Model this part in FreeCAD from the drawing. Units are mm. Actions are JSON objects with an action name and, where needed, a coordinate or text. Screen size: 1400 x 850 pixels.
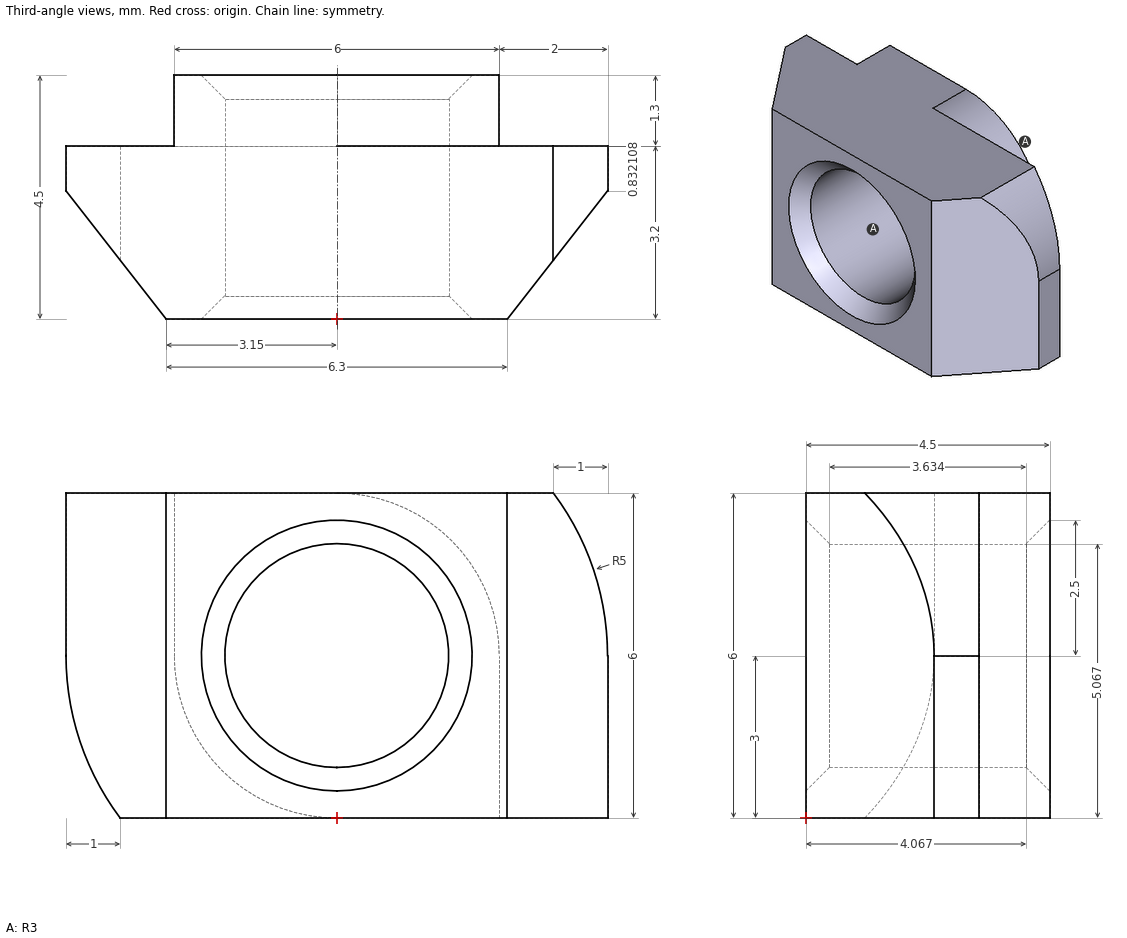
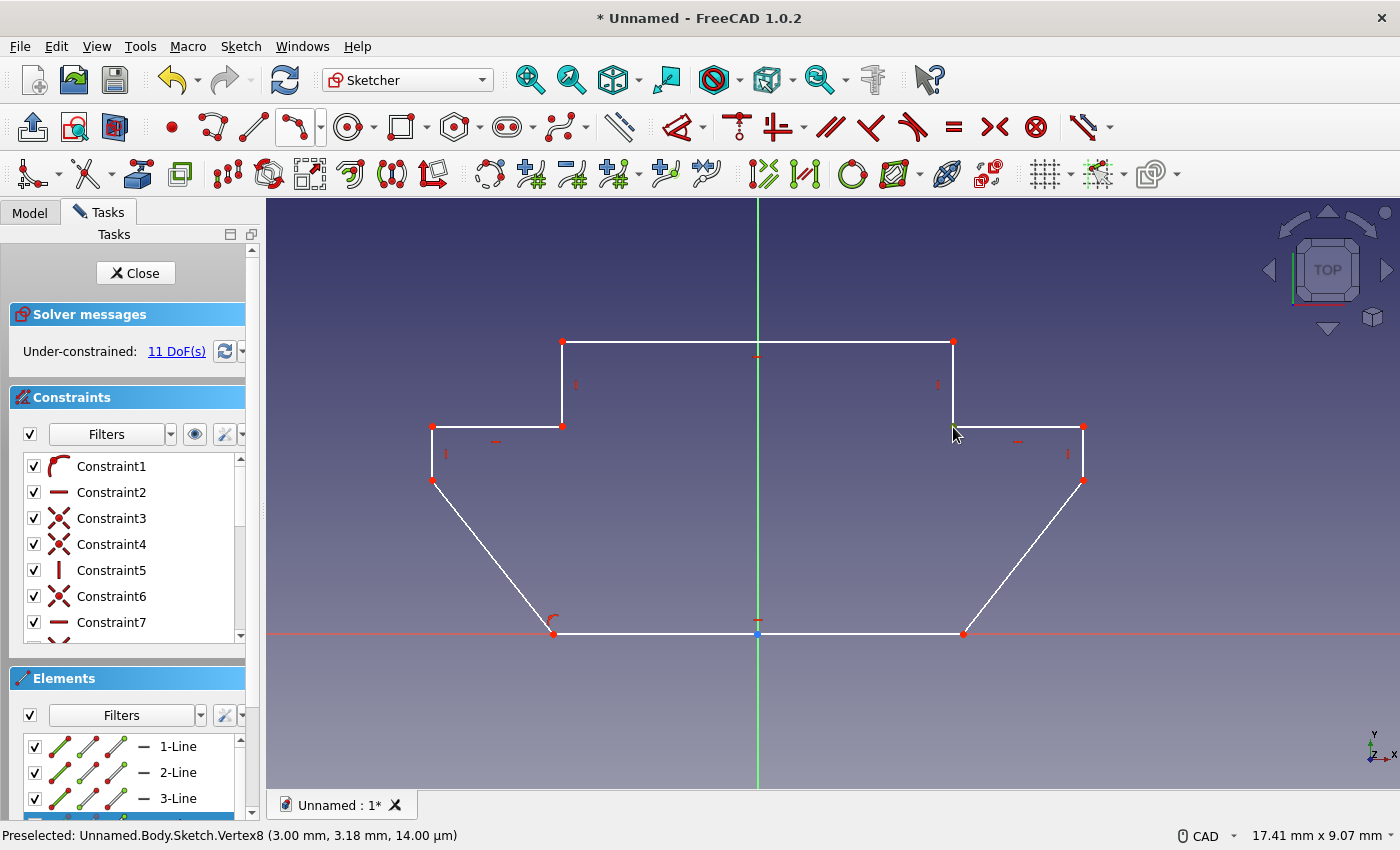
{"action": "left_click", "coordinate": [562, 427]}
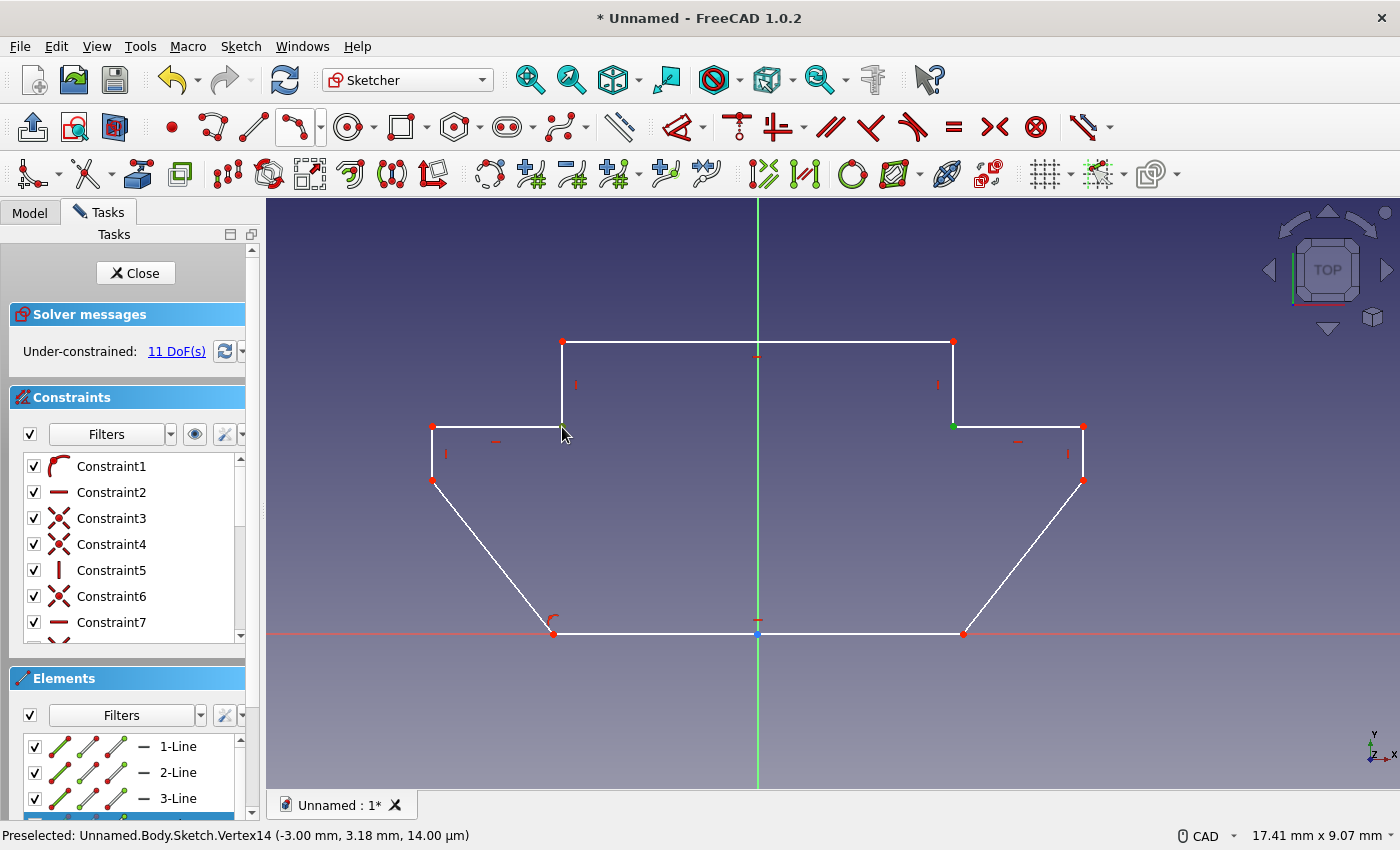
{"action": "left_click", "coordinate": [758, 723]}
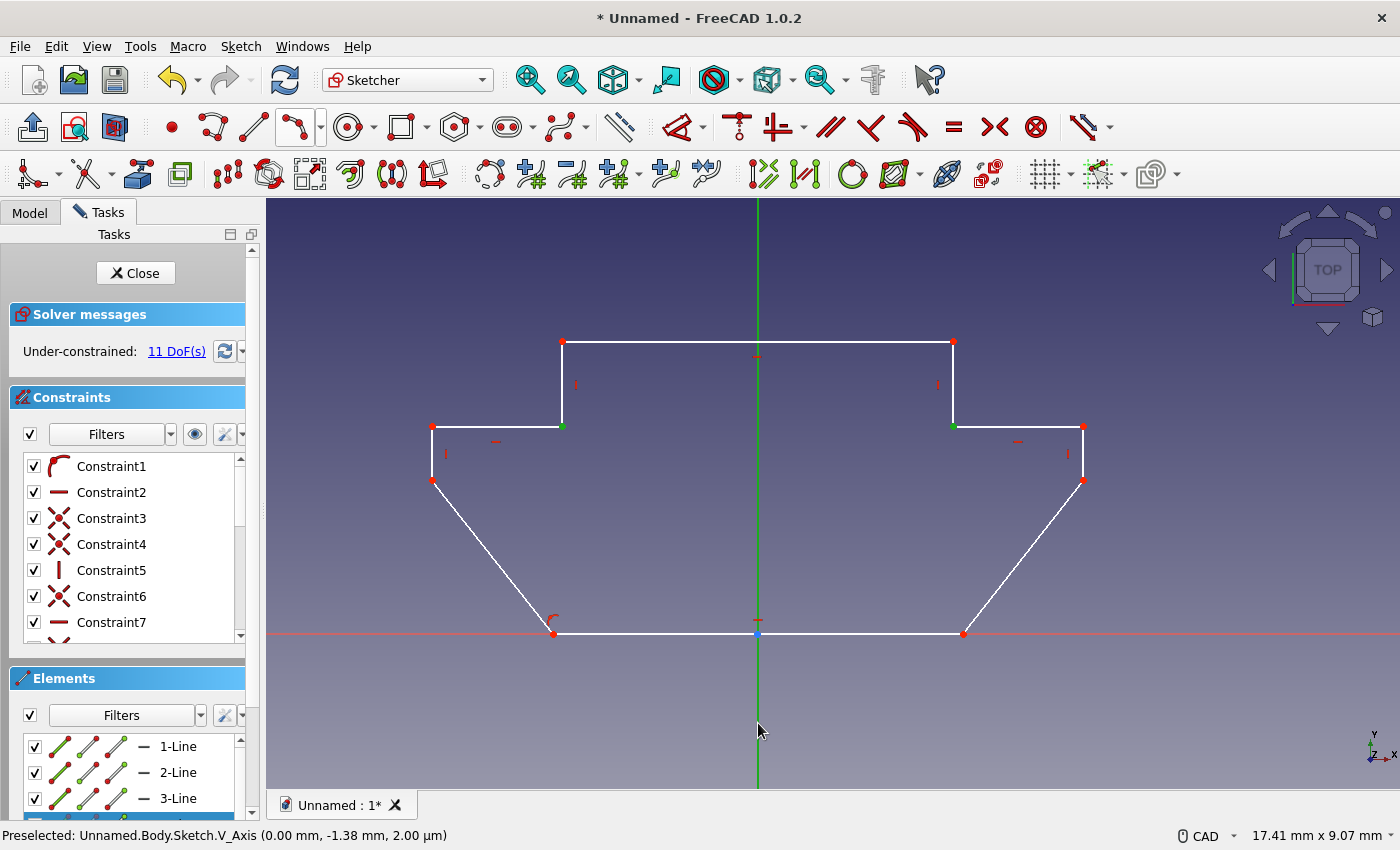
{"action": "left_click", "coordinate": [995, 128]}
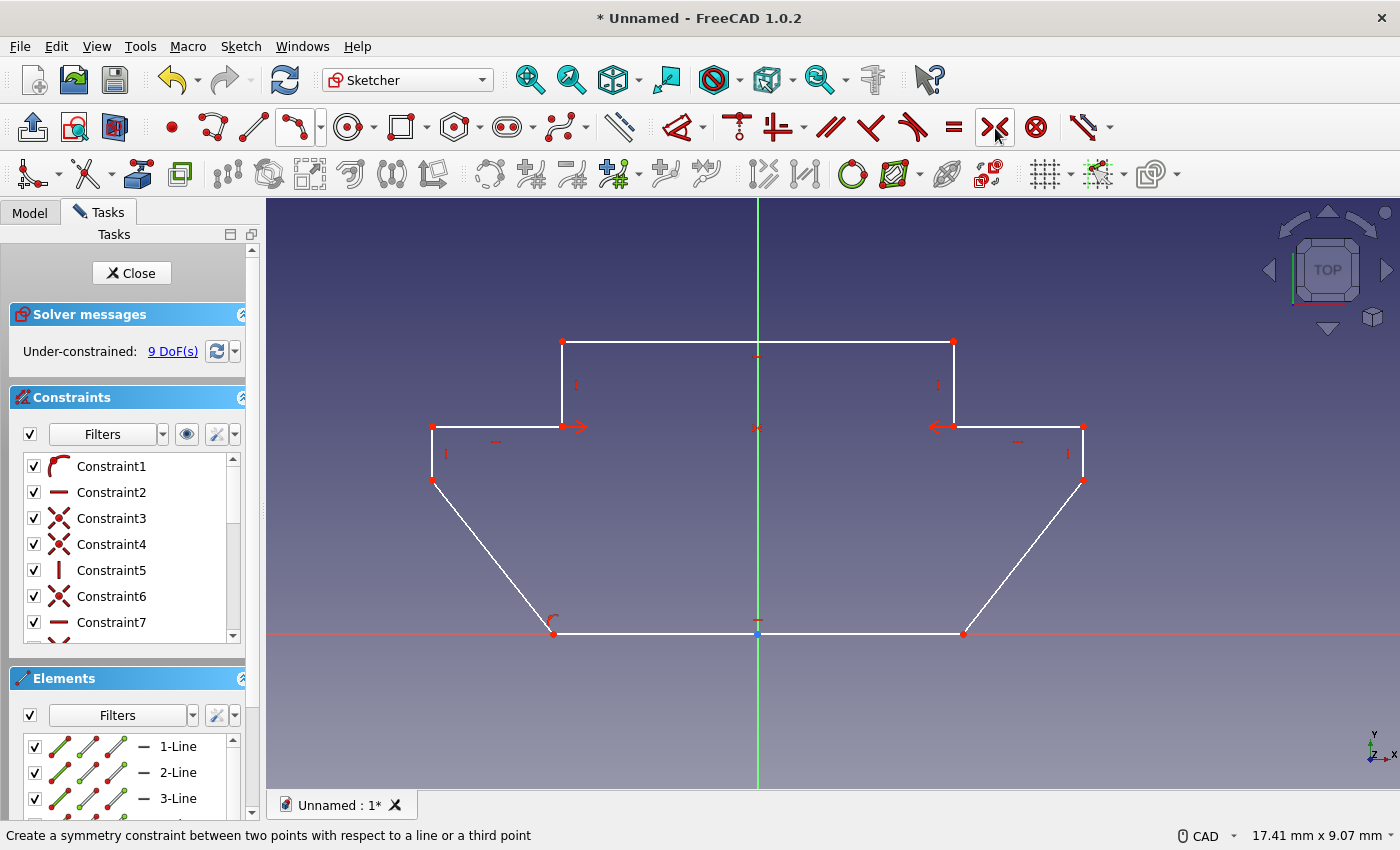
{"action": "left_click", "coordinate": [1083, 481]}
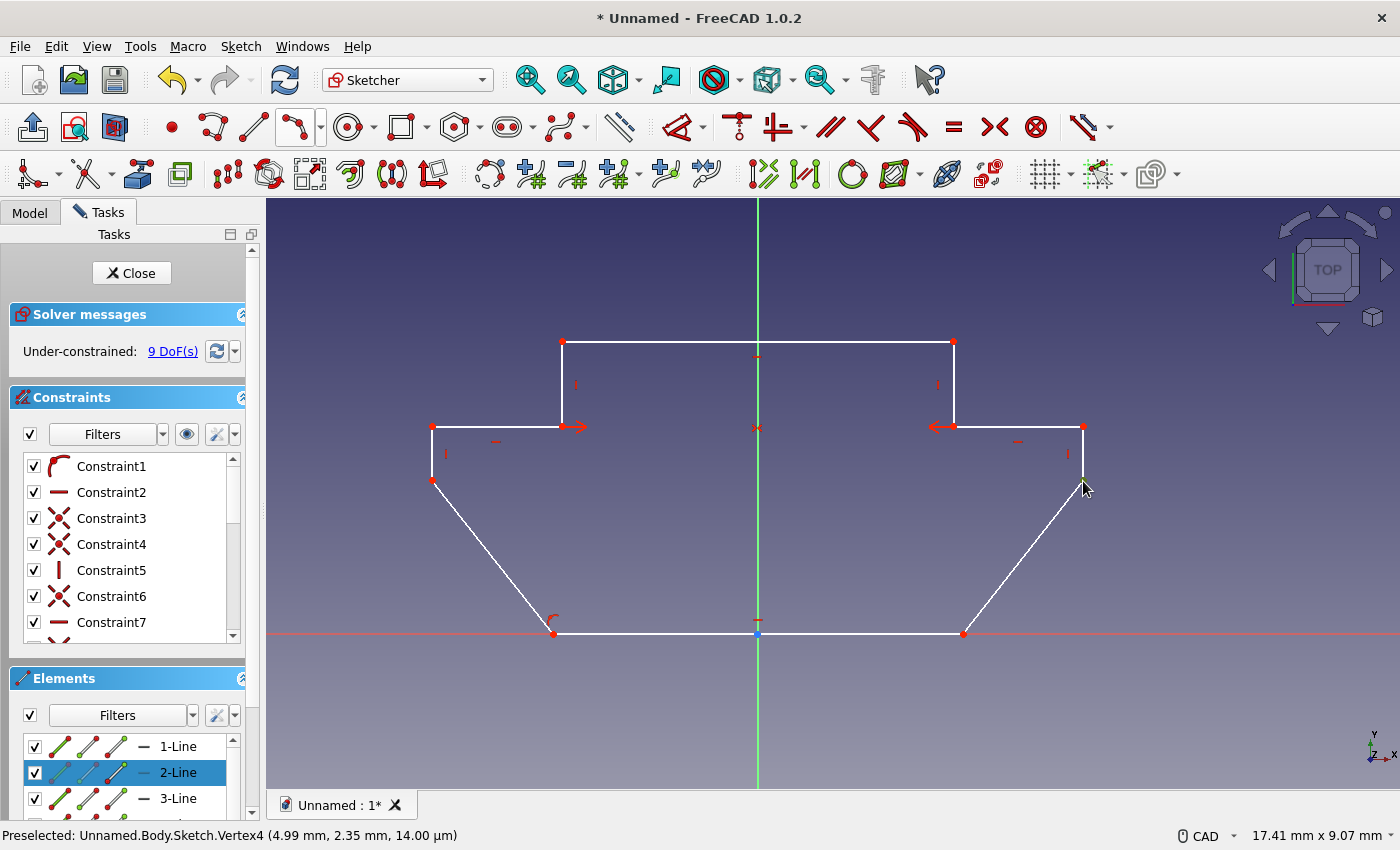
{"action": "left_click", "coordinate": [432, 481]}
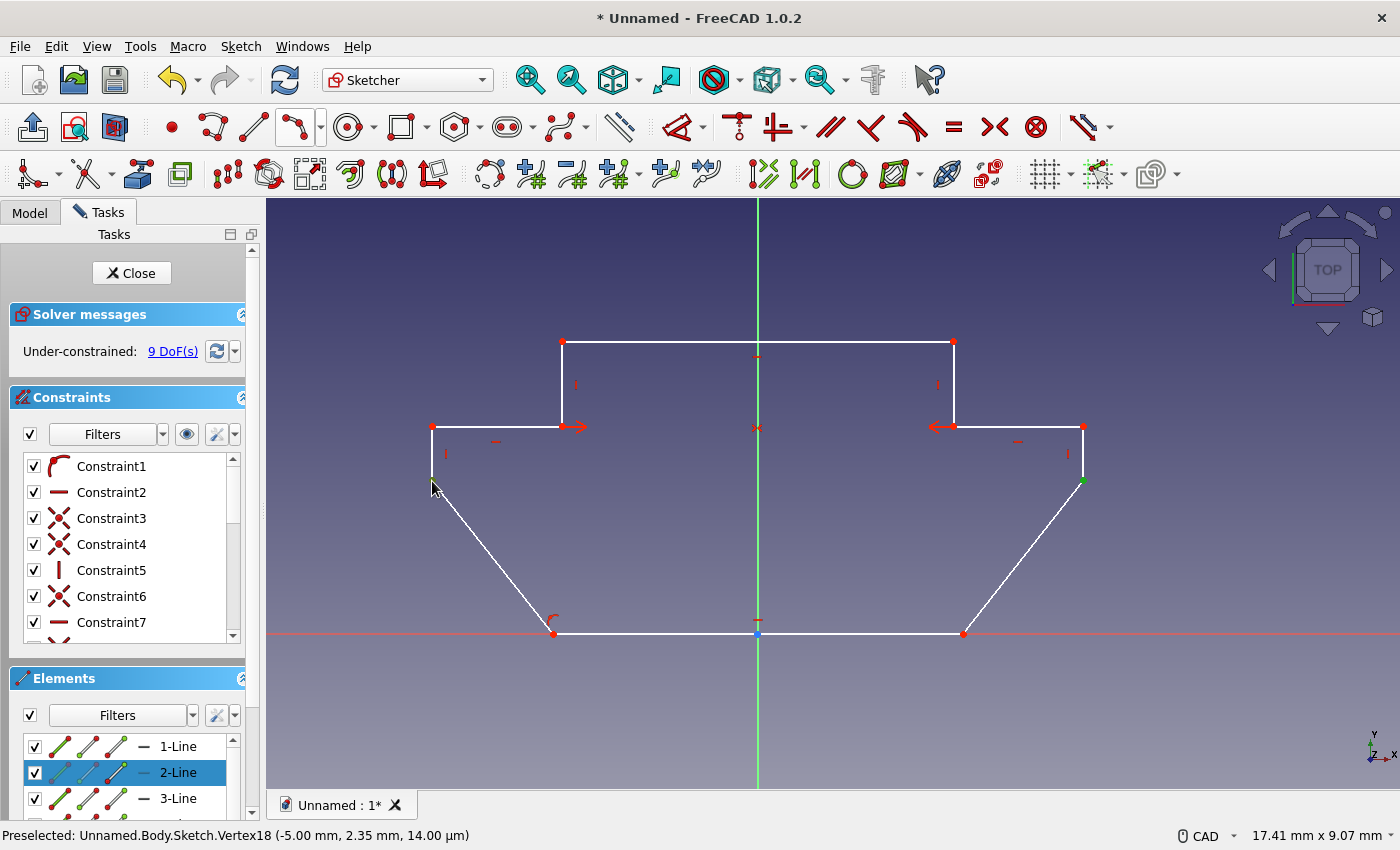
{"action": "left_click", "coordinate": [758, 723]}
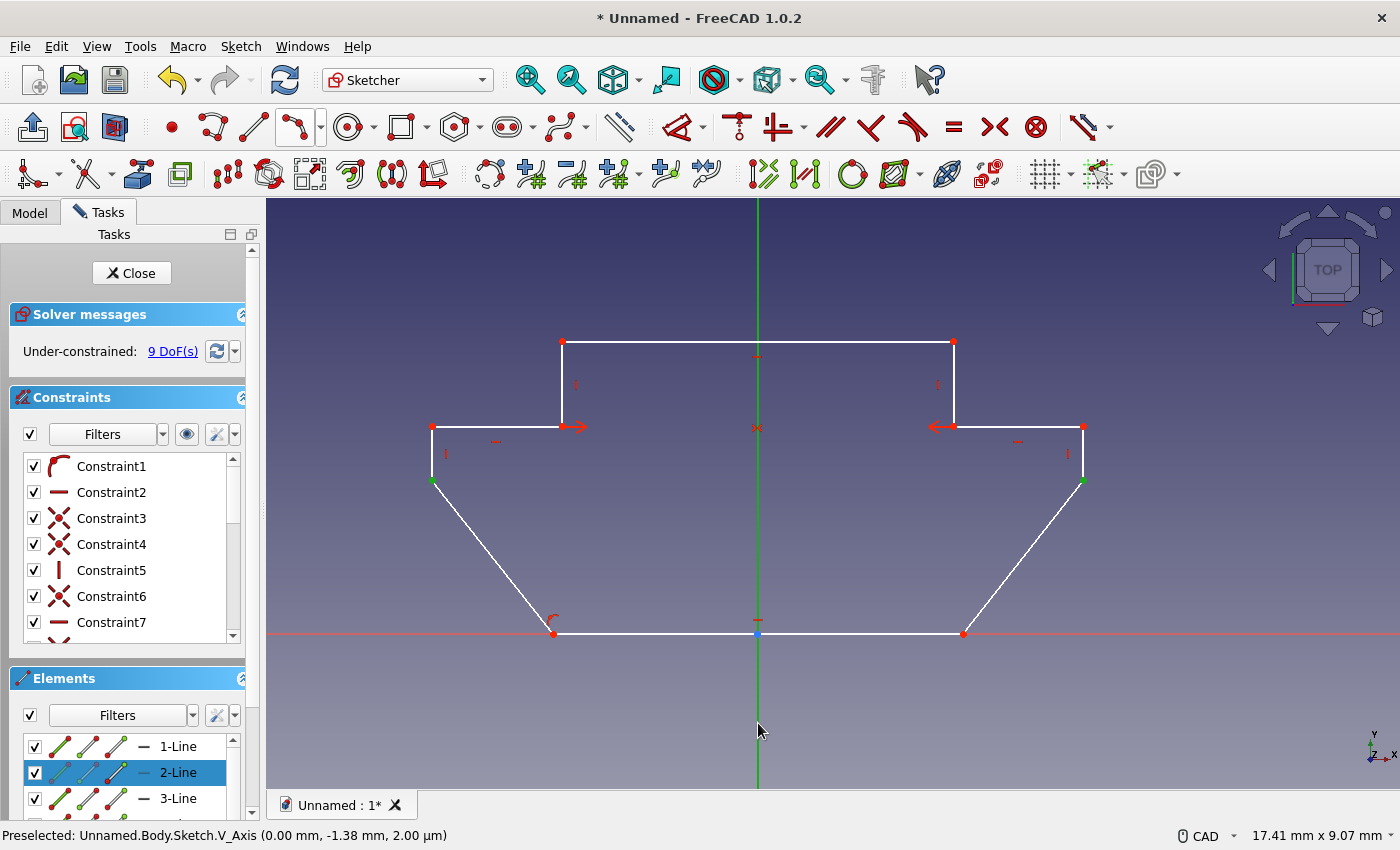
{"action": "left_click", "coordinate": [995, 128]}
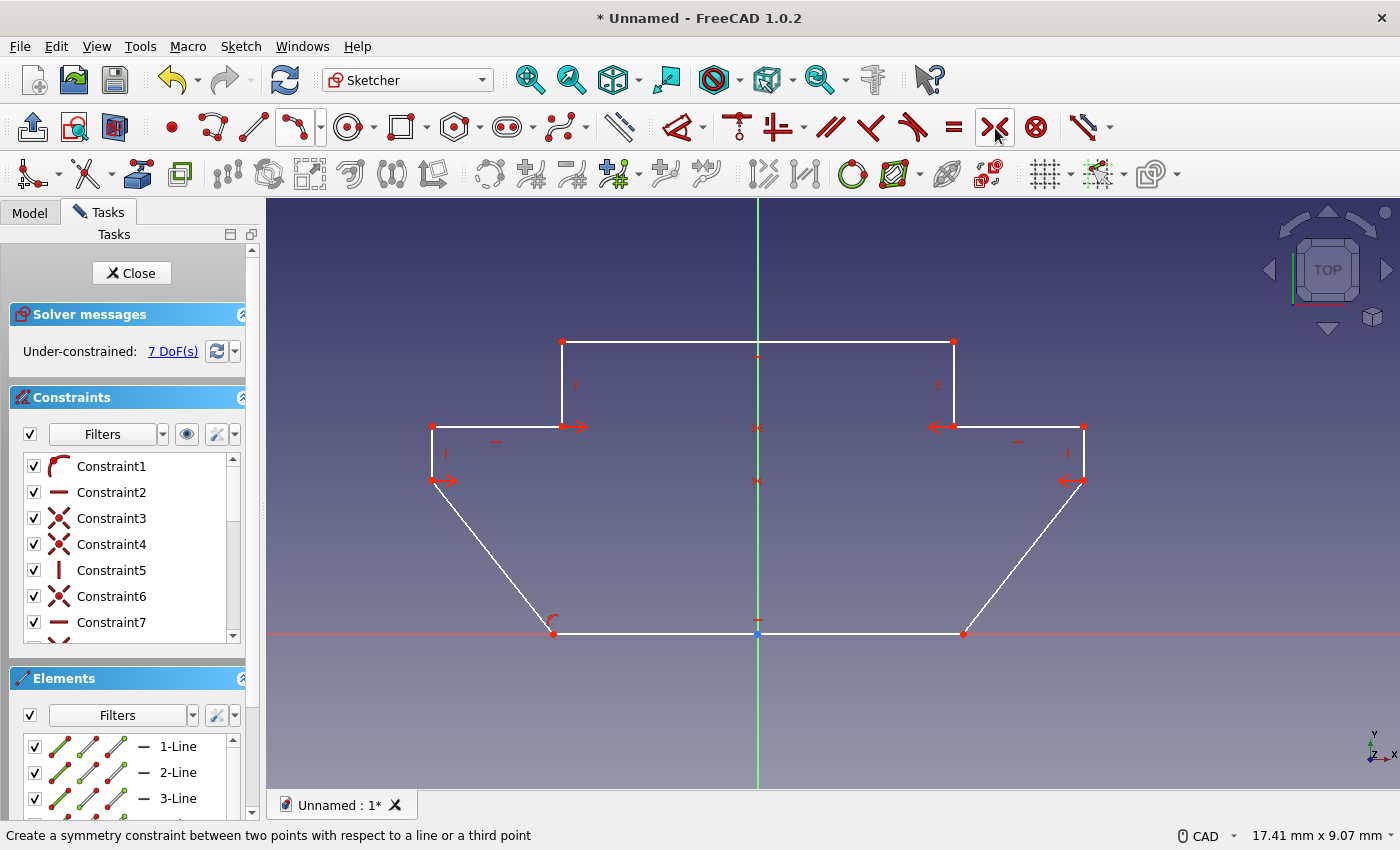
{"action": "left_click", "coordinate": [676, 128]}